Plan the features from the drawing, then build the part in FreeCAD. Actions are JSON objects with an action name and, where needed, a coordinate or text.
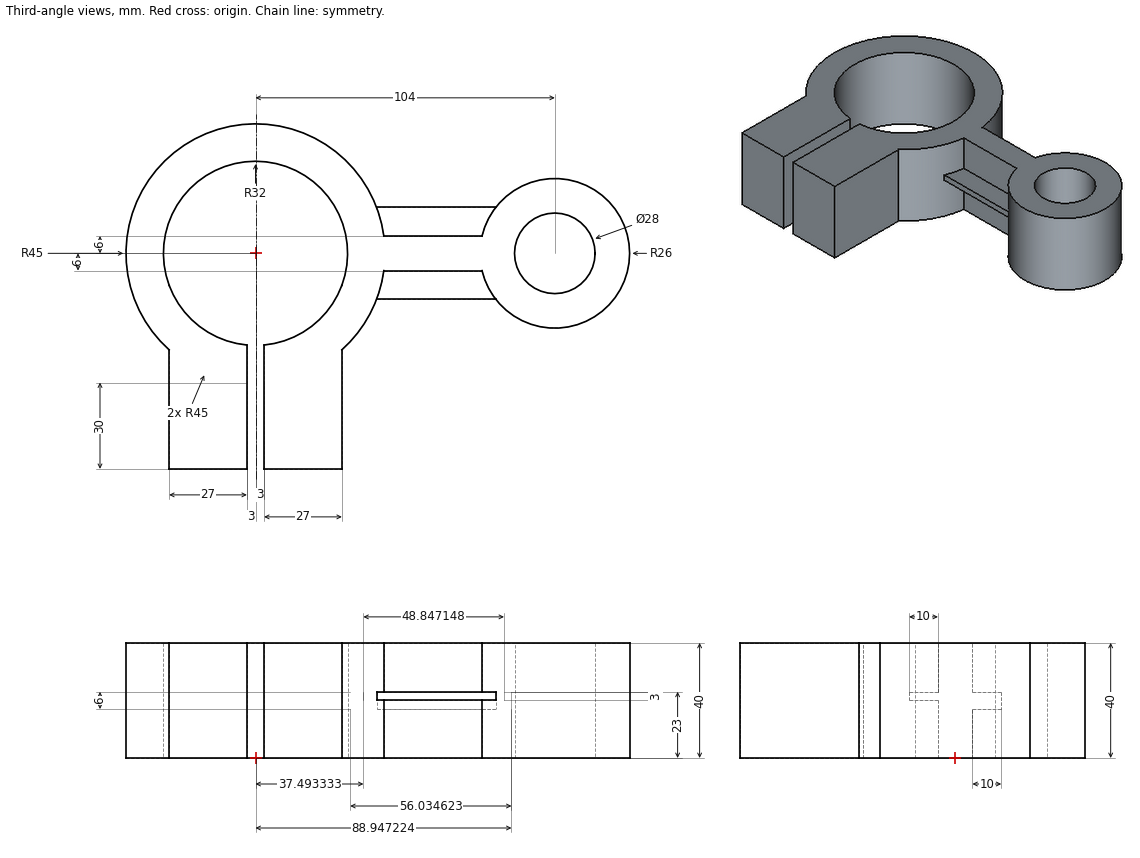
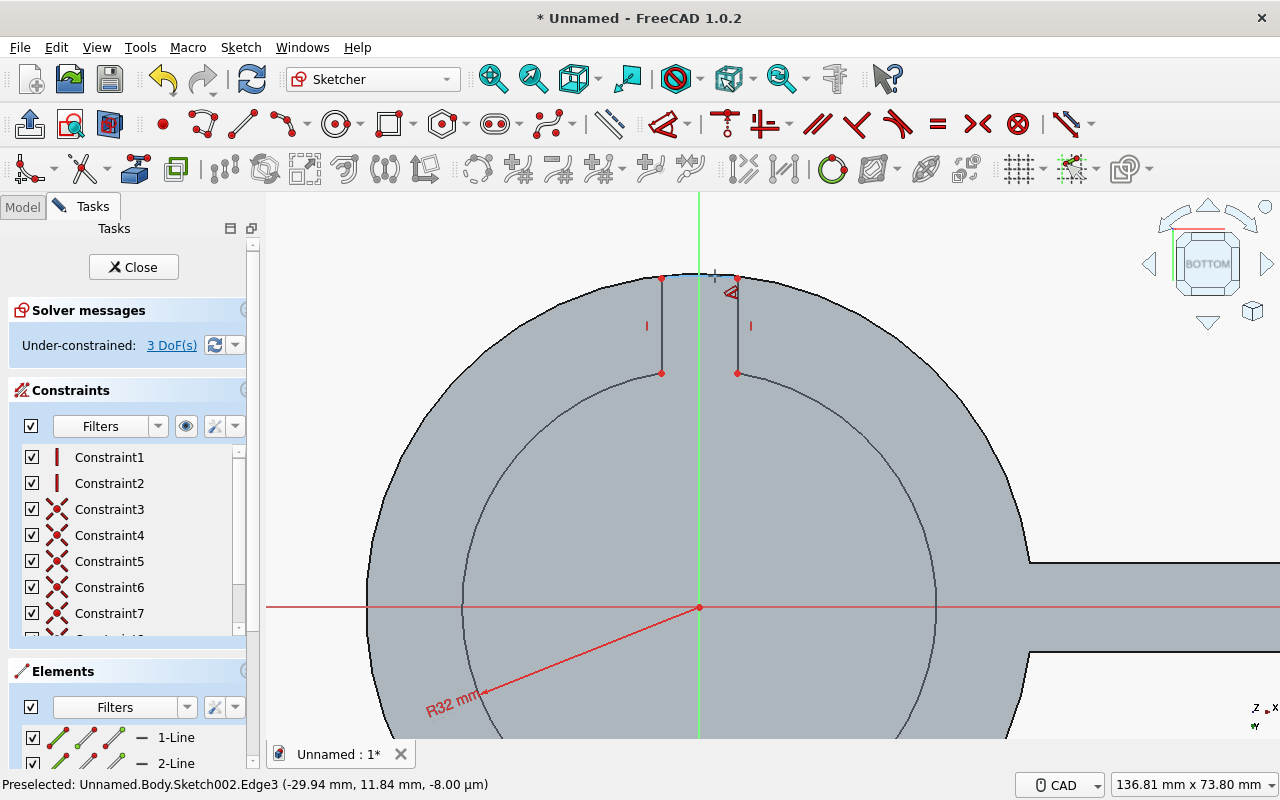
{"action": "left_click", "coordinate": [715, 276]}
{"action": "left_click", "coordinate": [717, 244]}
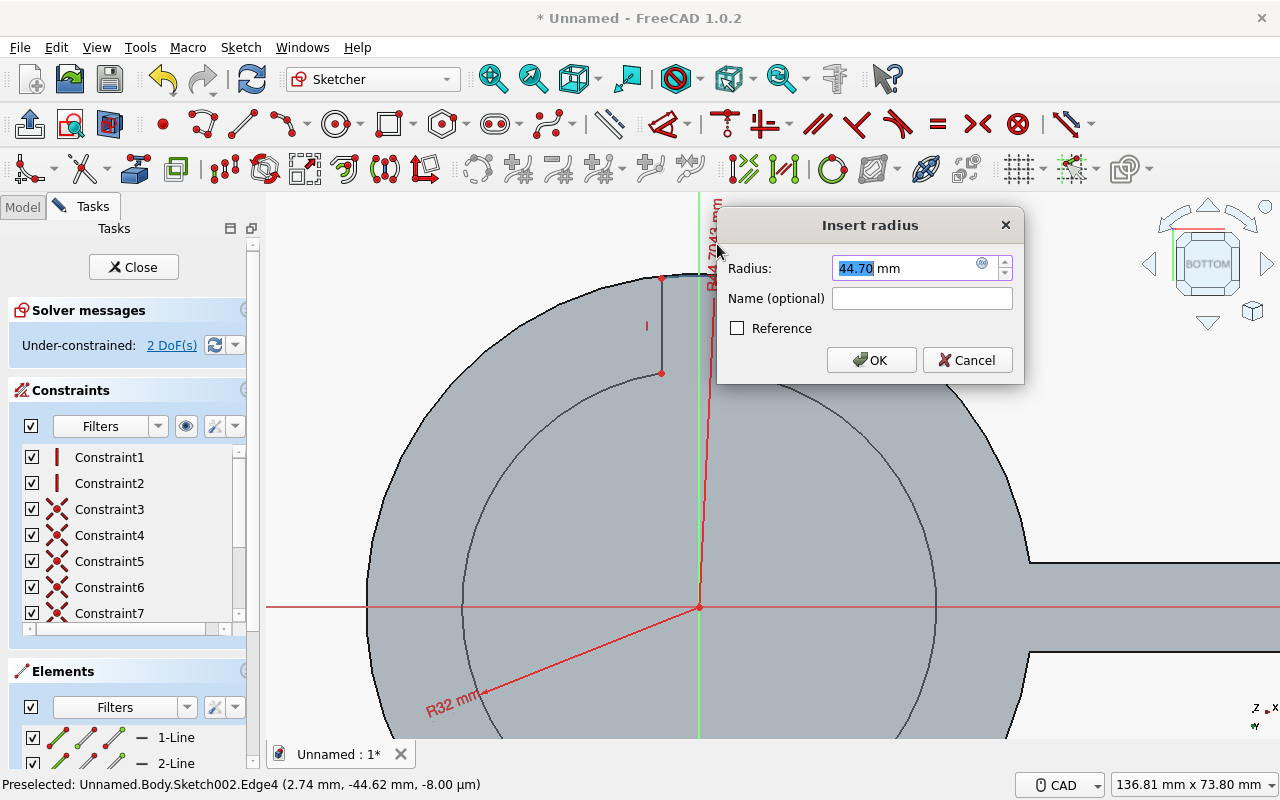
{"action": "type", "text": "45"}
{"action": "key", "text": "Return"}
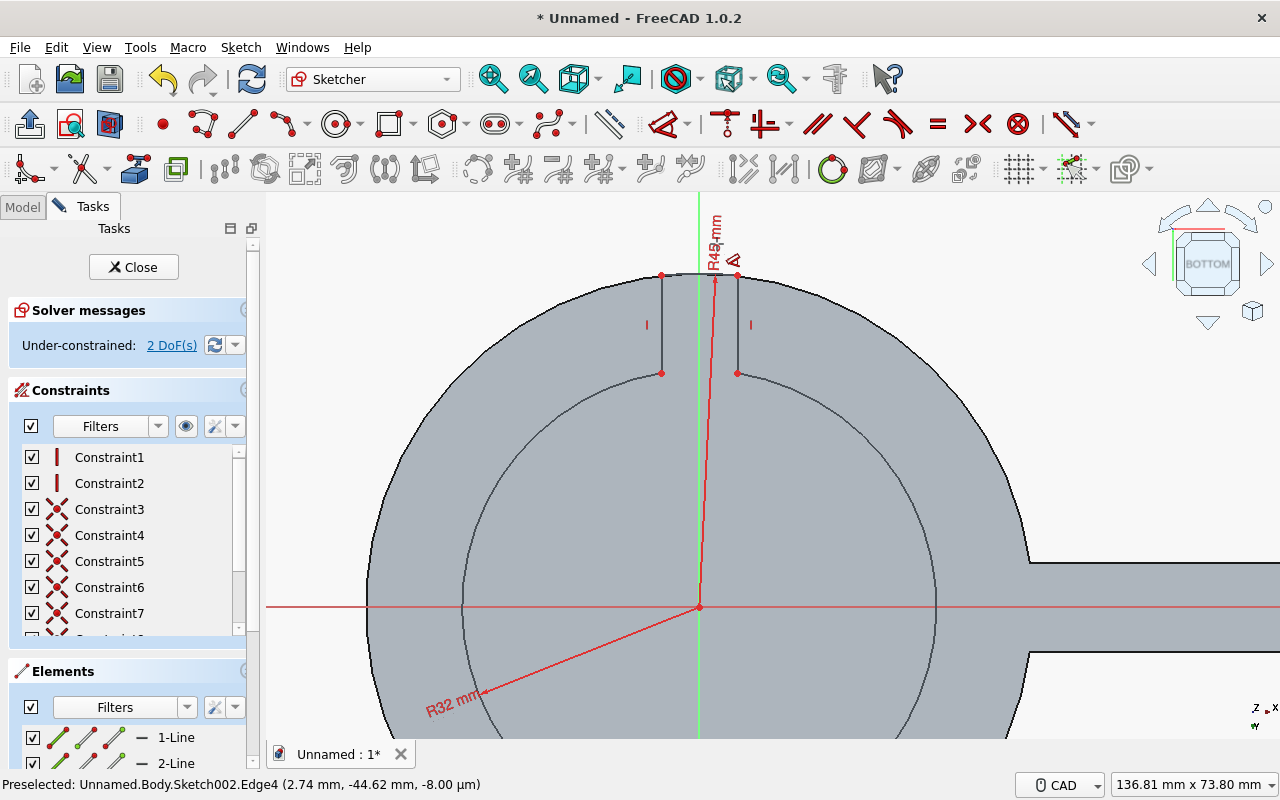
{"action": "scroll", "coordinate": [738, 276], "scroll_direction": "up", "scroll_amount": 3}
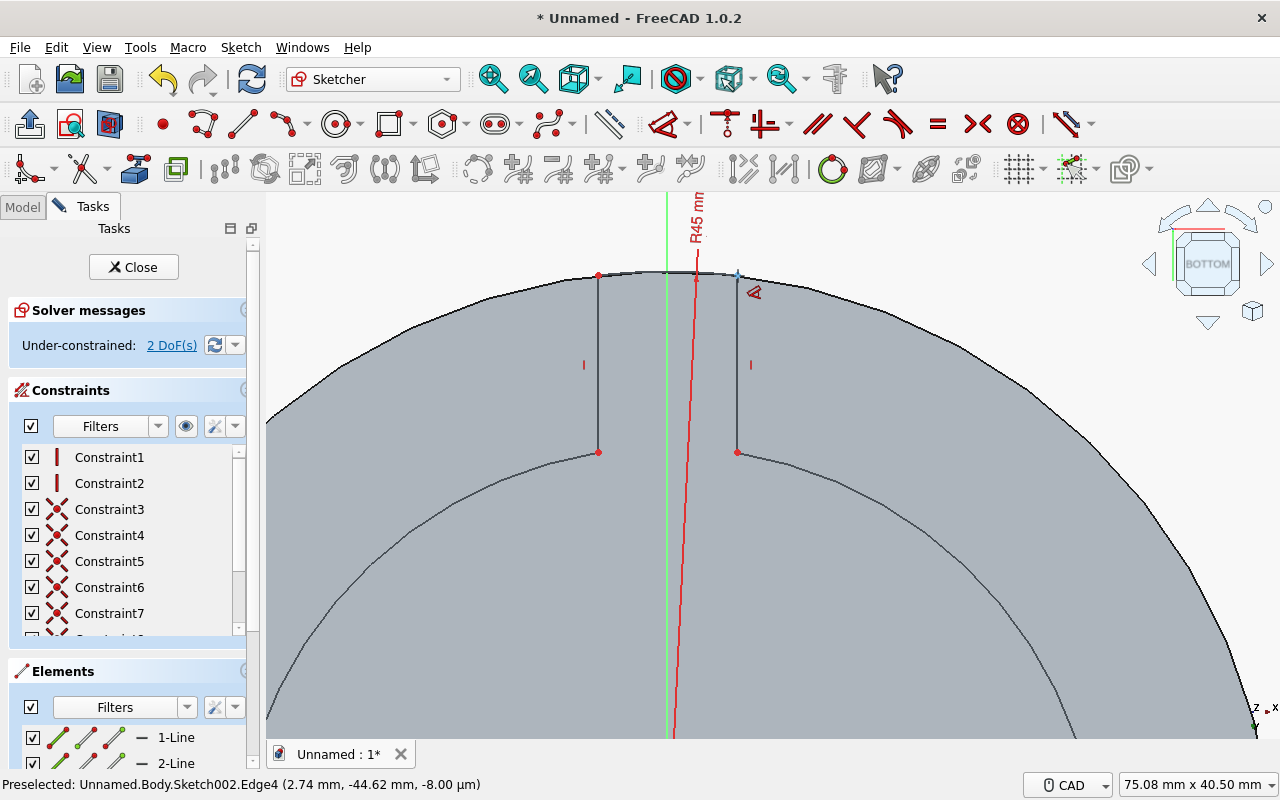
{"action": "left_click", "coordinate": [737, 276]}
{"action": "left_click", "coordinate": [702, 242]}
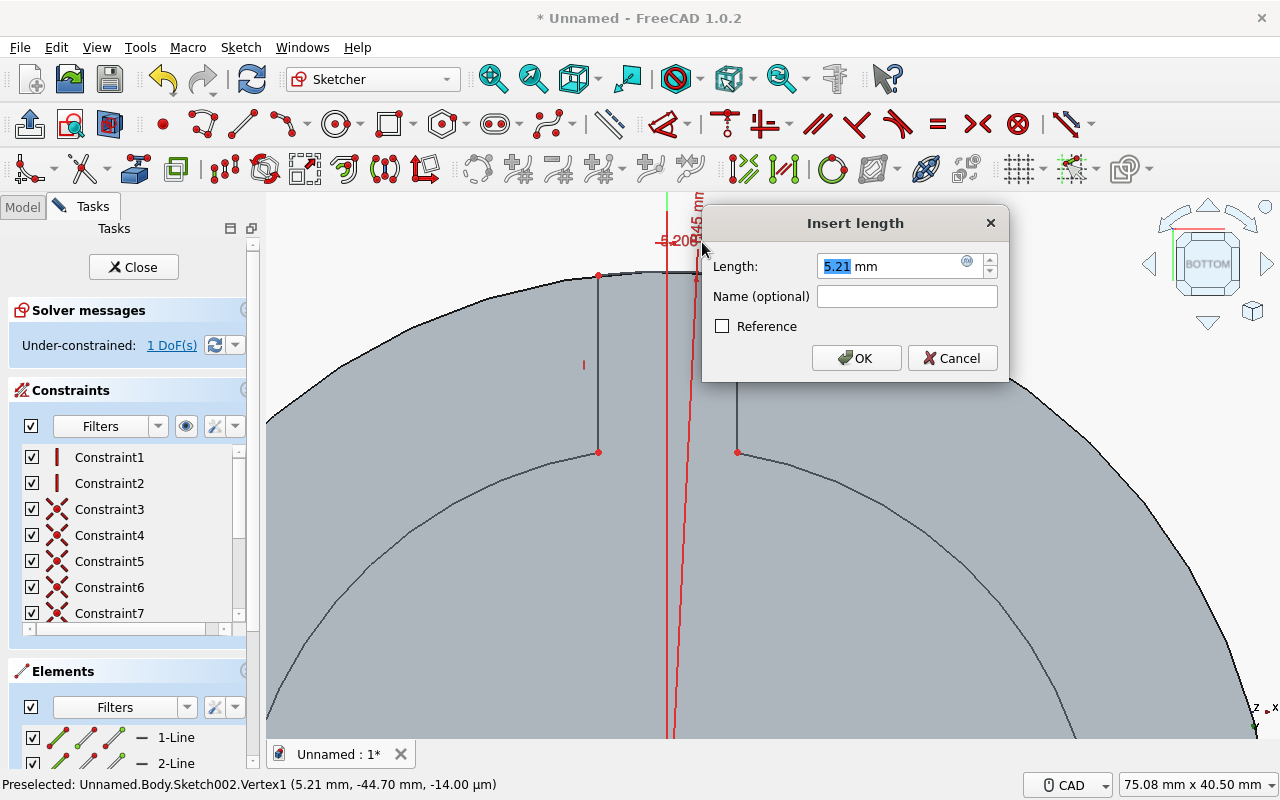
{"action": "type", "text": "3"}
{"action": "key", "text": "Return"}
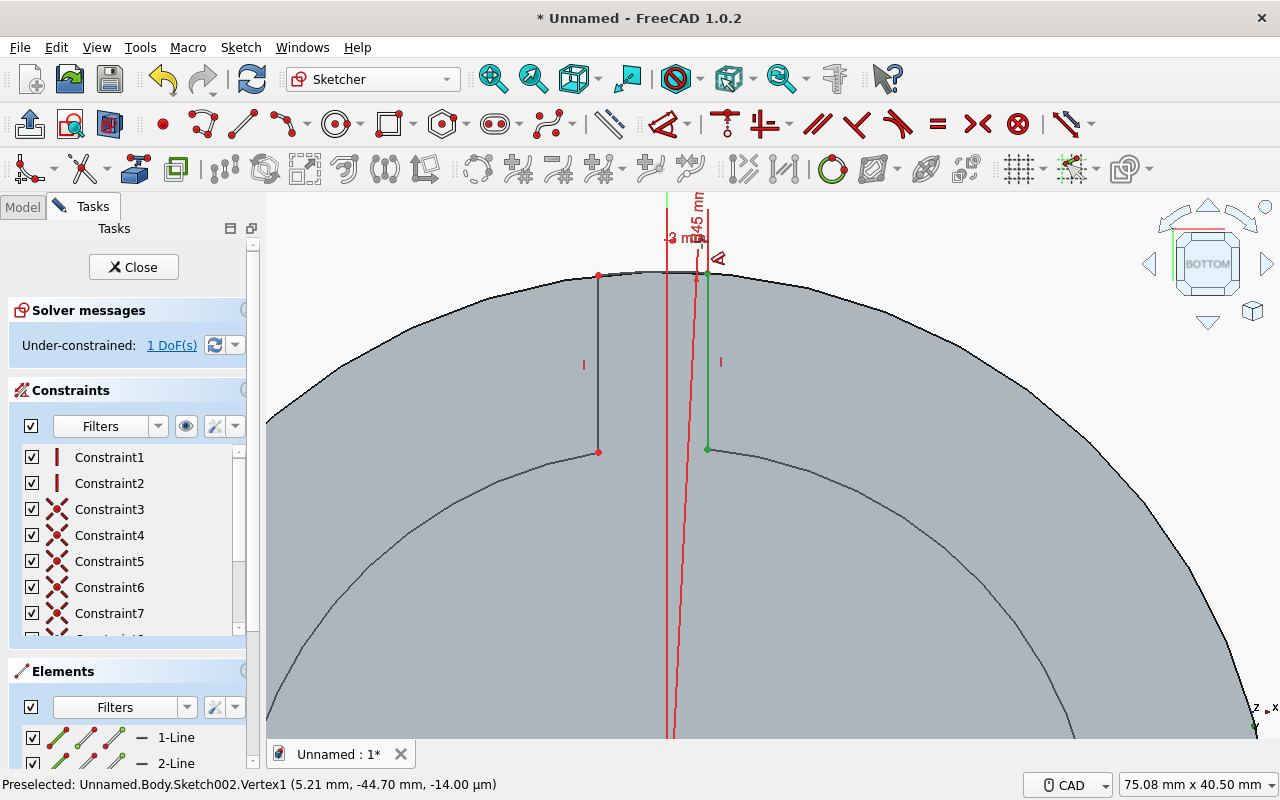
{"action": "left_click", "coordinate": [598, 453]}
{"action": "left_click", "coordinate": [633, 419]}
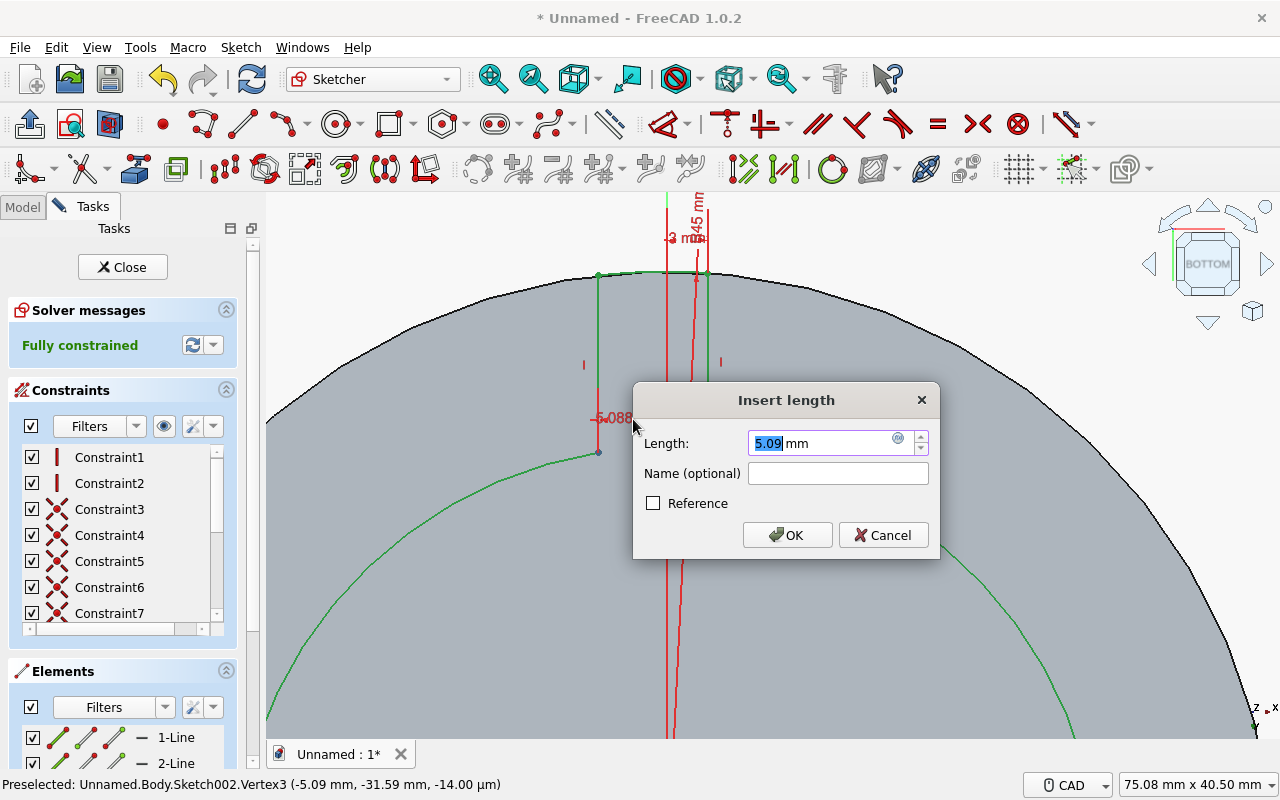
{"action": "type", "text": "3"}
{"action": "key", "text": "Return"}
{"action": "key", "text": "Escape"}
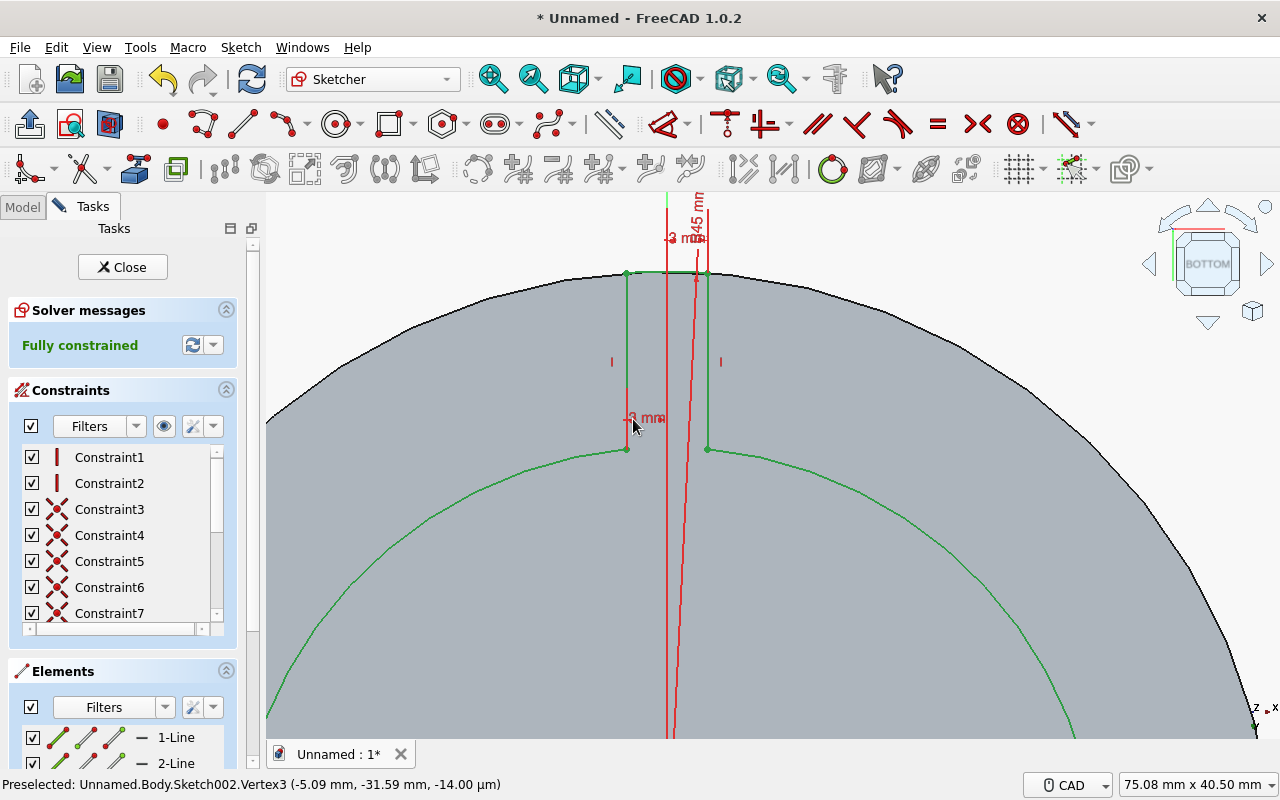
{"action": "left_click", "coordinate": [123, 267]}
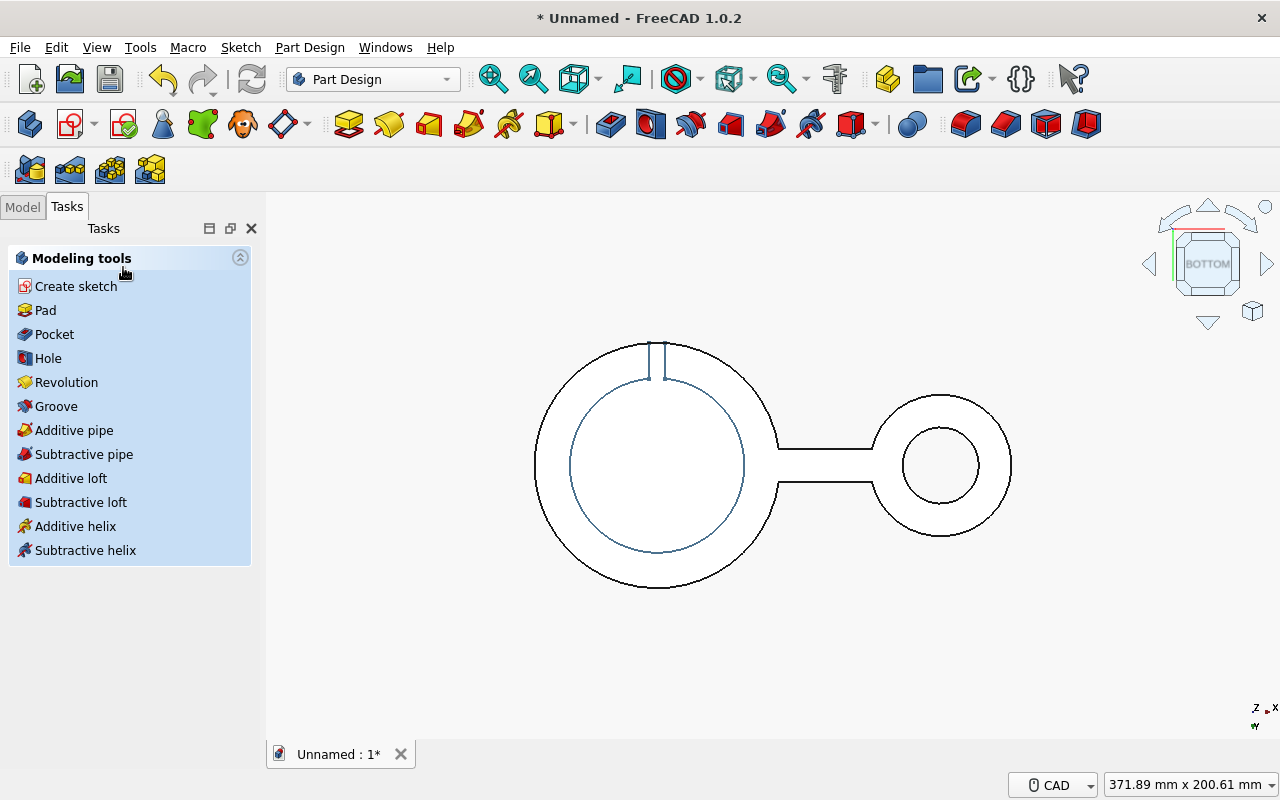
{"action": "left_click", "coordinate": [612, 124]}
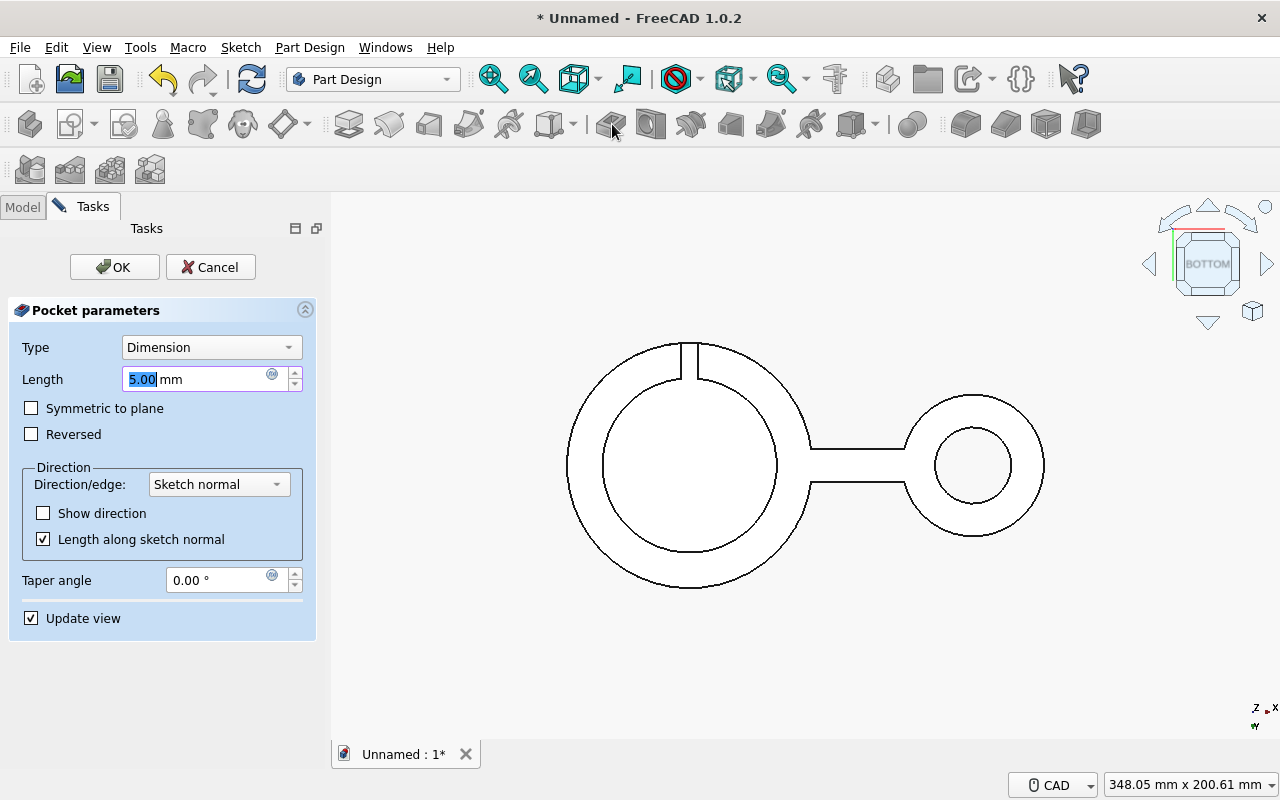
{"action": "type", "text": "40"}
{"action": "key", "text": "Tab"}